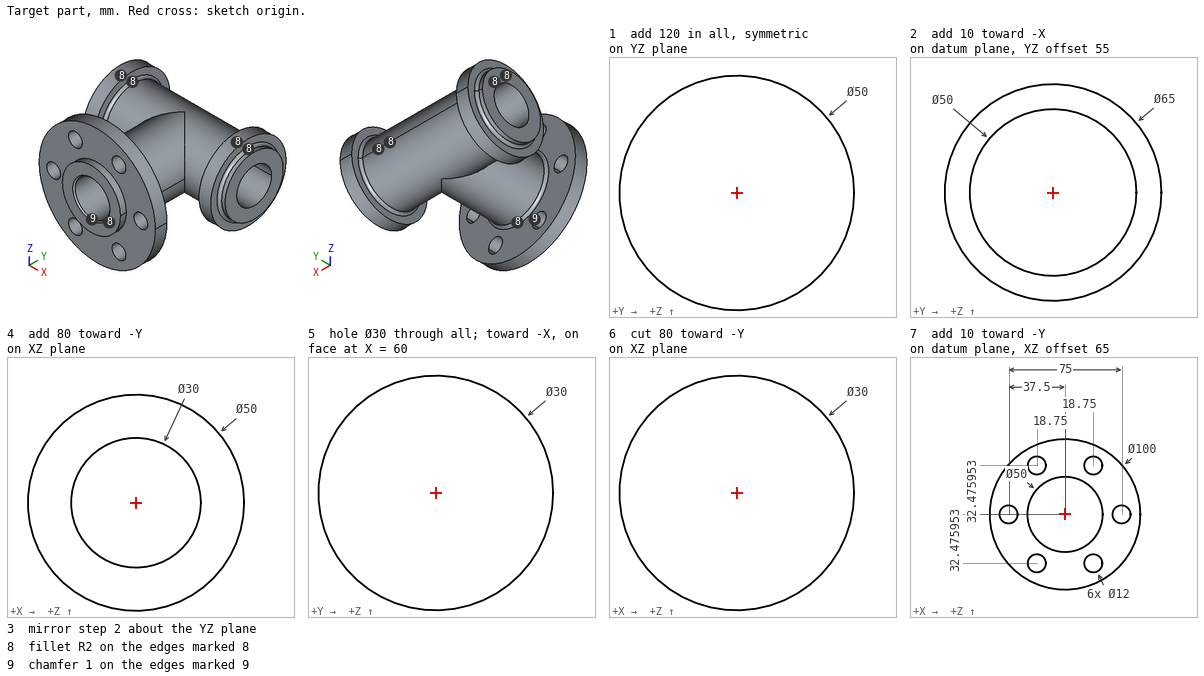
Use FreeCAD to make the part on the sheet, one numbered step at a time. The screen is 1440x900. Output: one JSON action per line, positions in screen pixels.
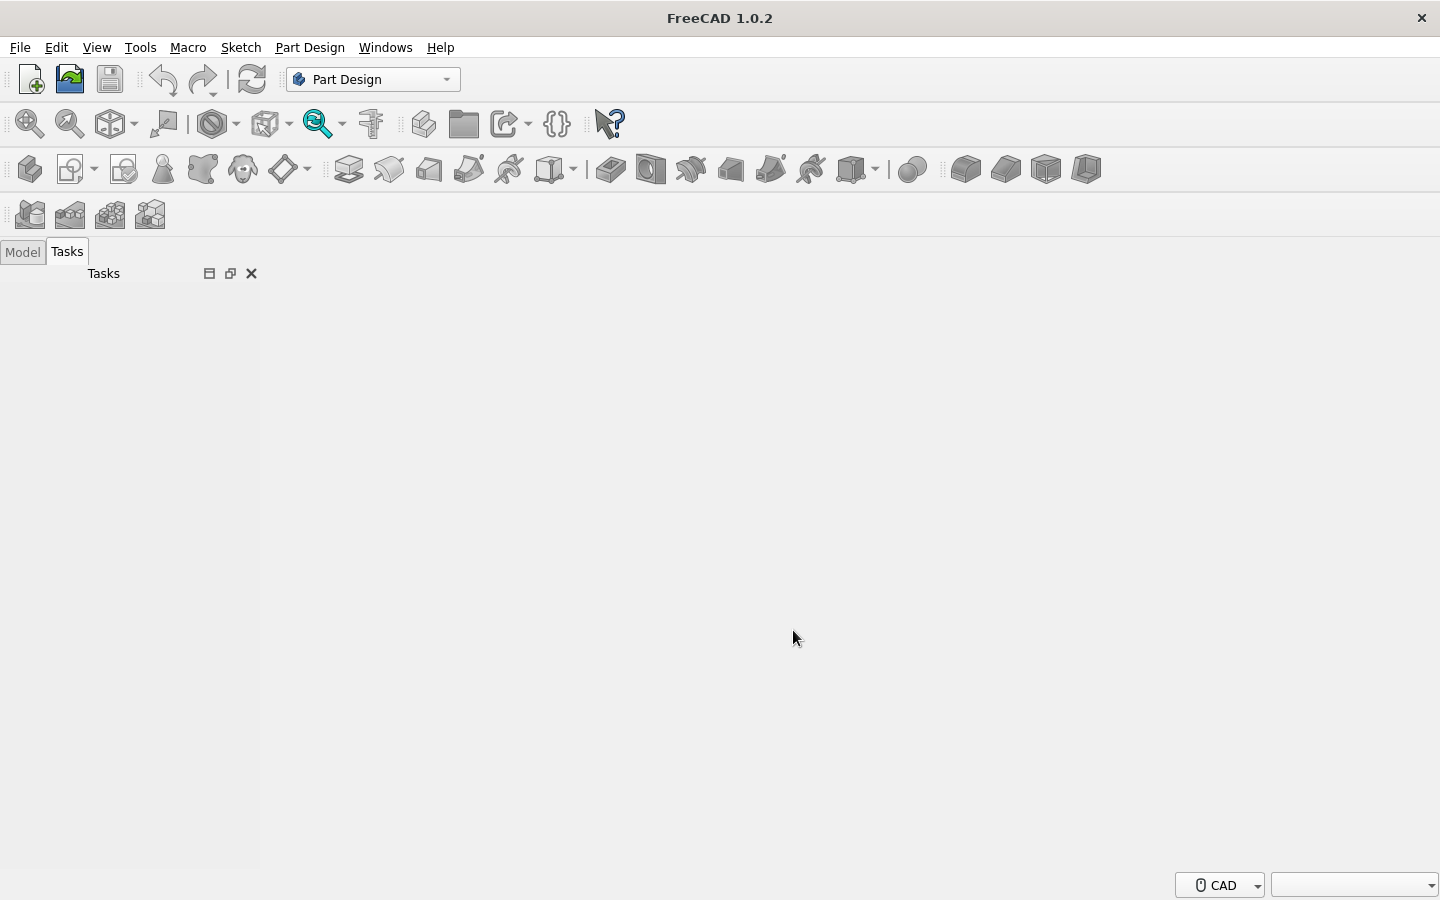
{"action": "key", "text": "ctrl+n"}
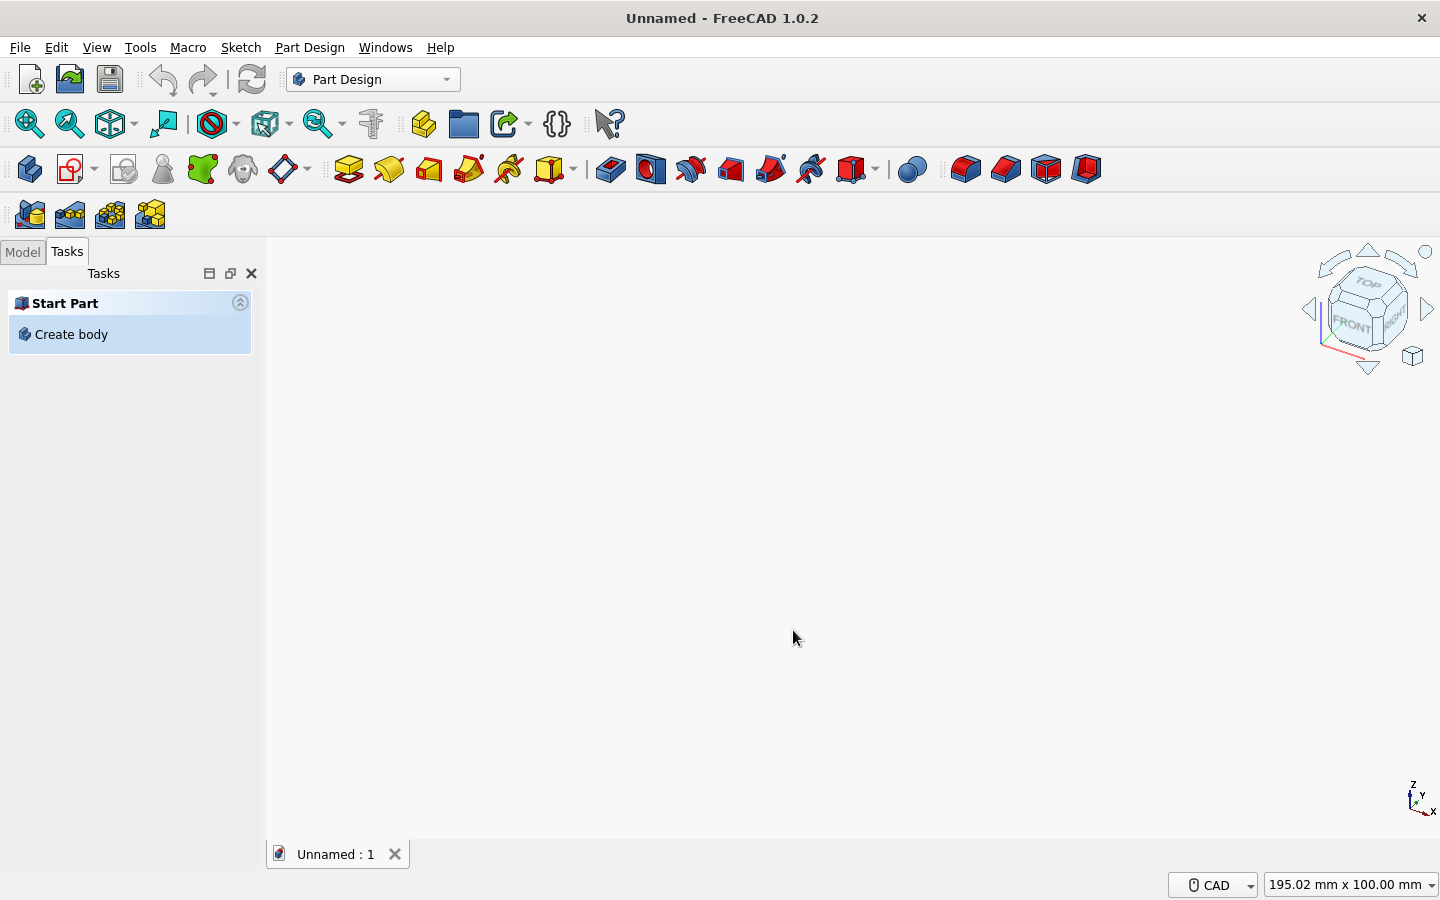
{"action": "left_click", "coordinate": [70, 170]}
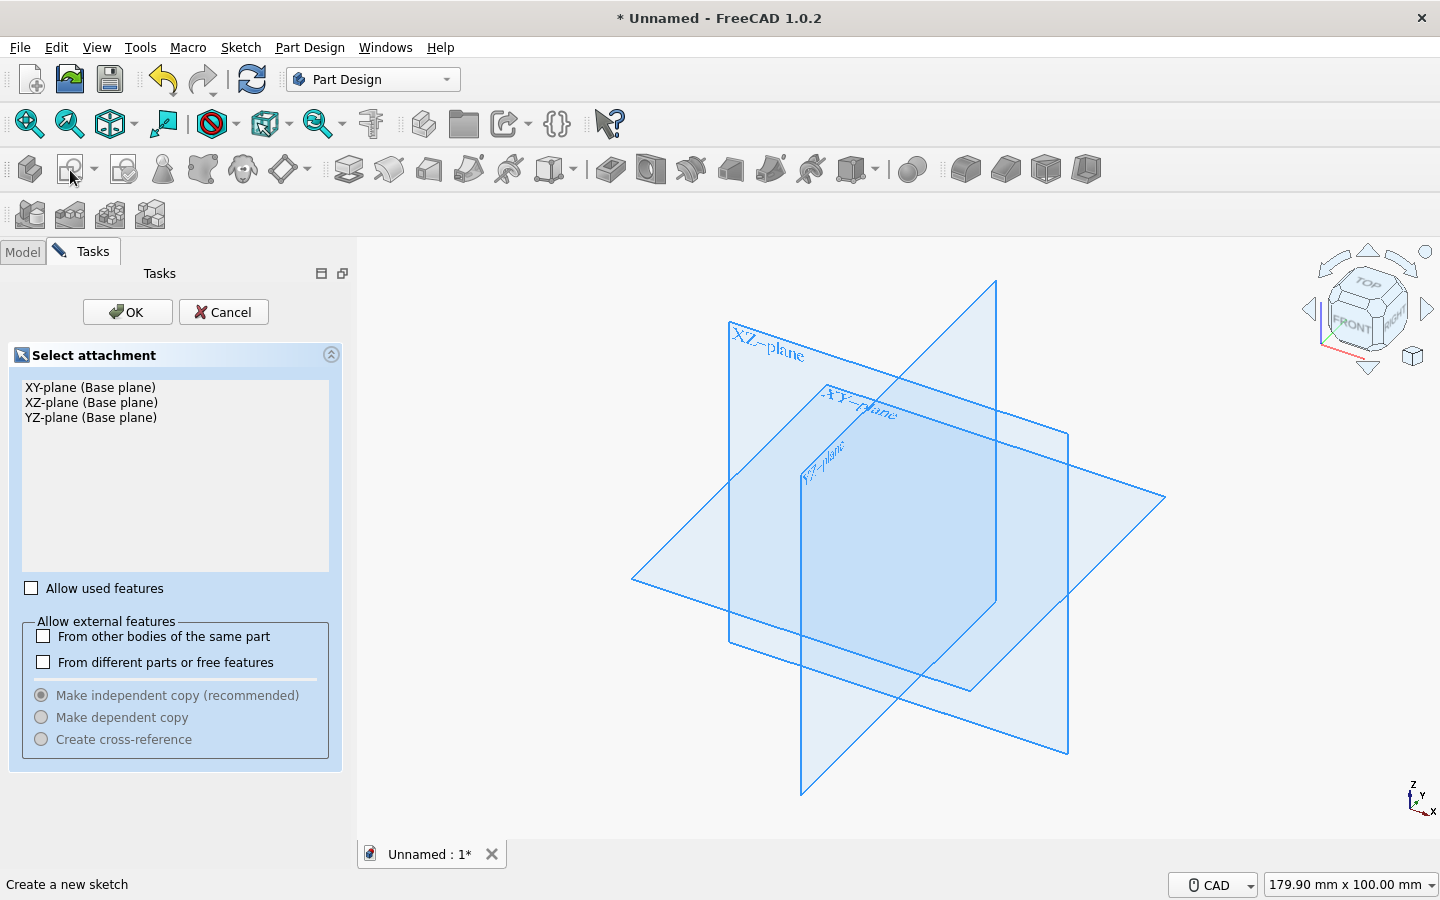
{"action": "left_click", "coordinate": [82, 418]}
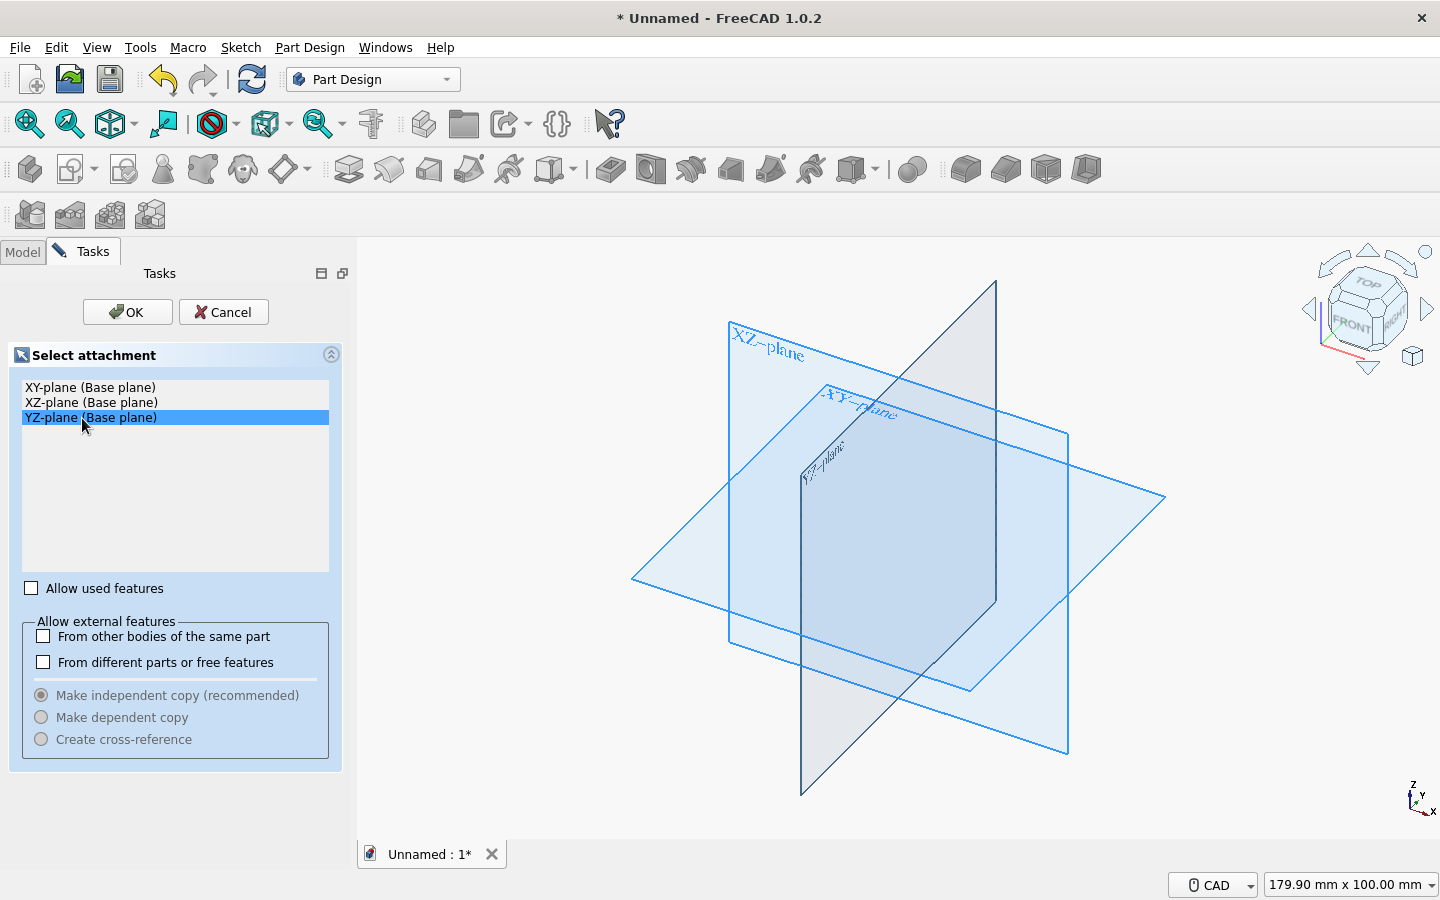
{"action": "left_click", "coordinate": [128, 312]}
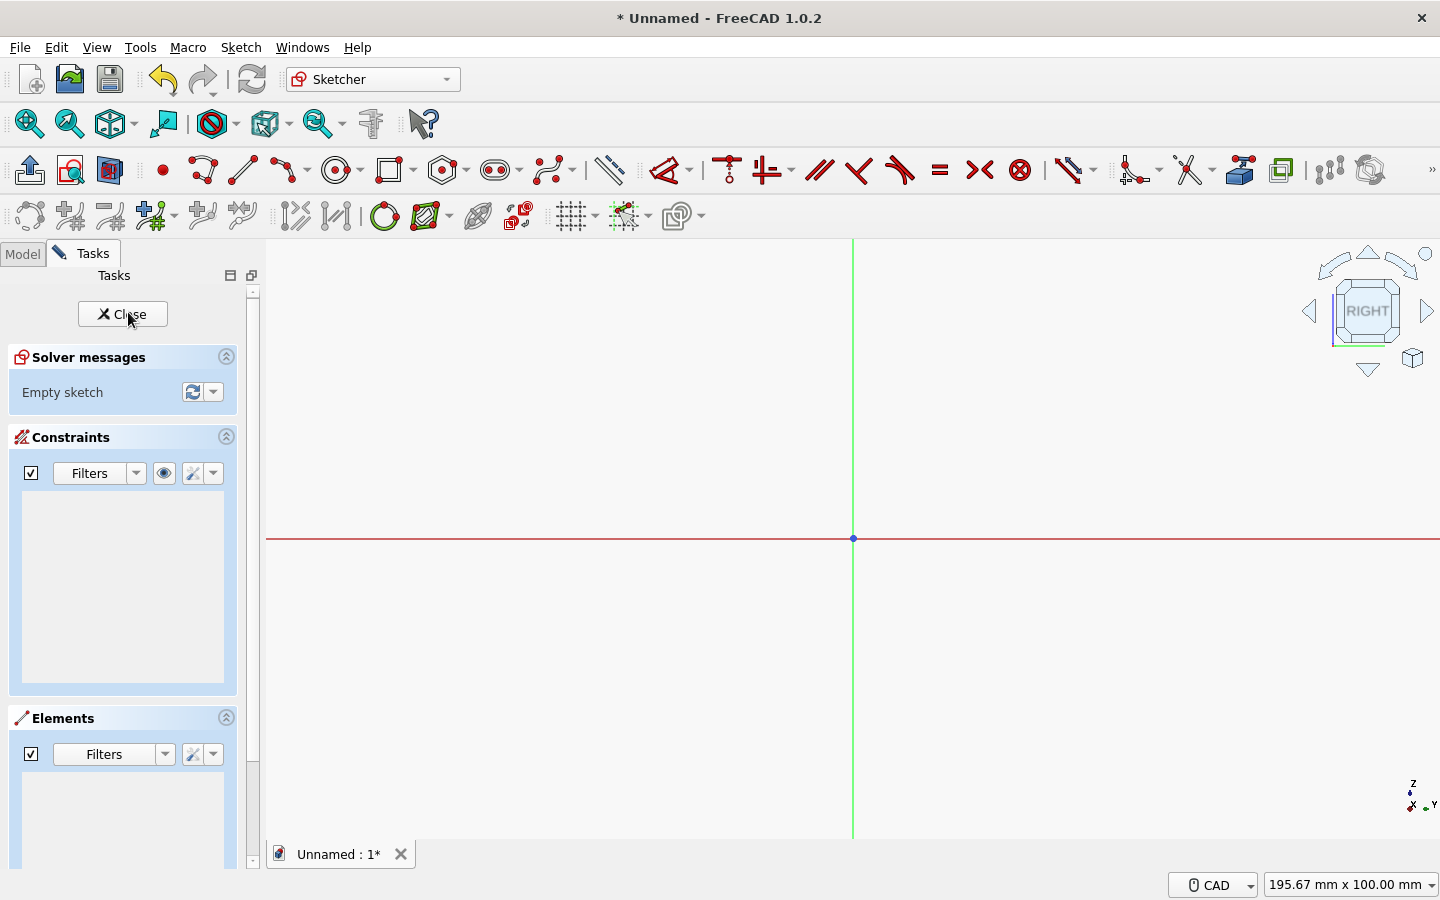
{"action": "left_click", "coordinate": [336, 170]}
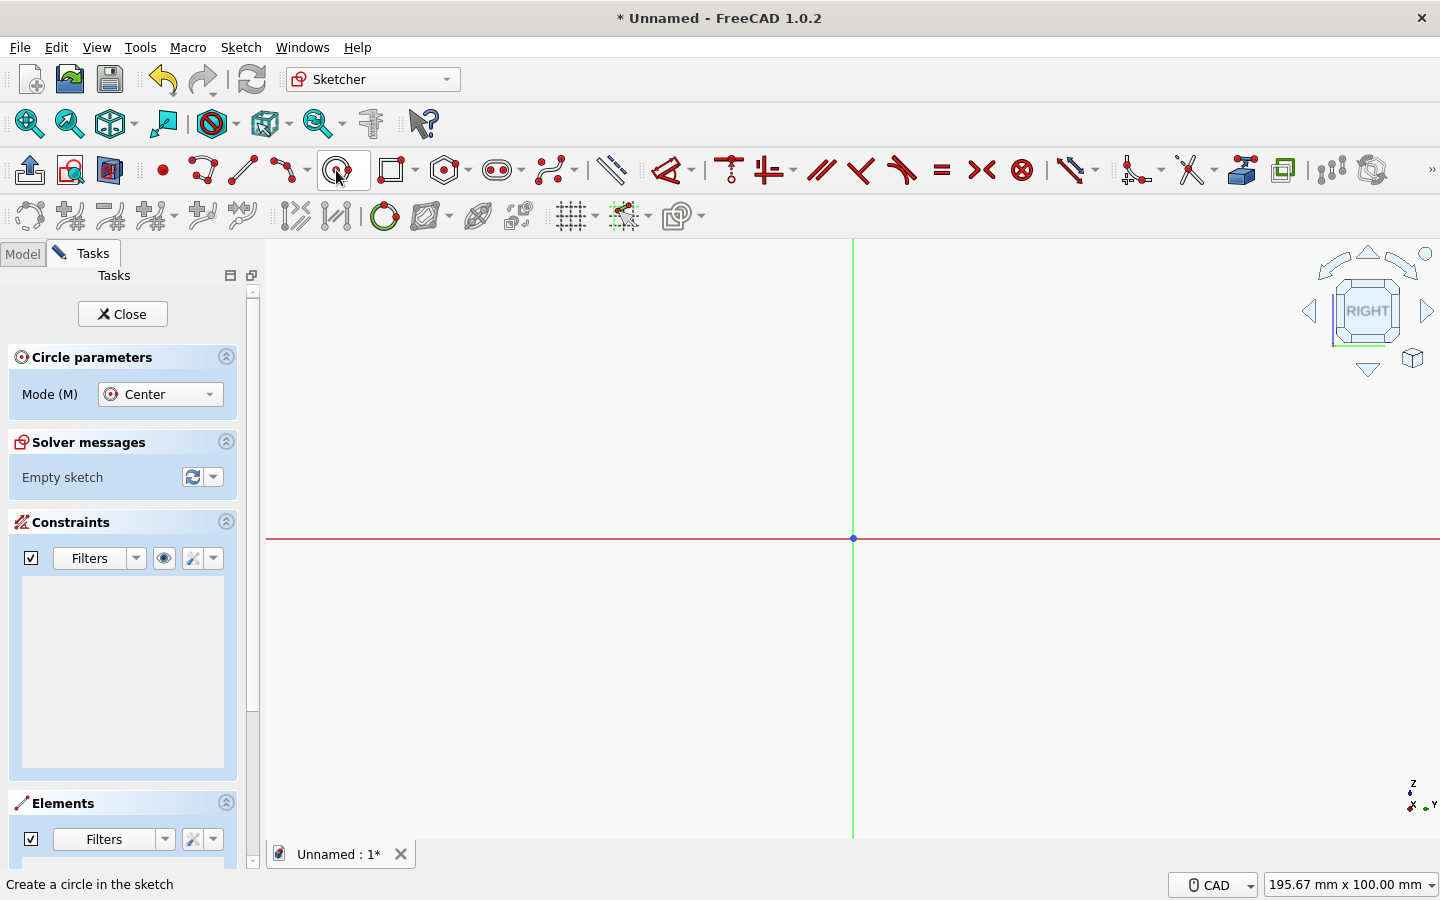
{"action": "left_click", "coordinate": [853, 539]}
{"action": "left_click", "coordinate": [959, 433]}
{"action": "key", "text": "Escape"}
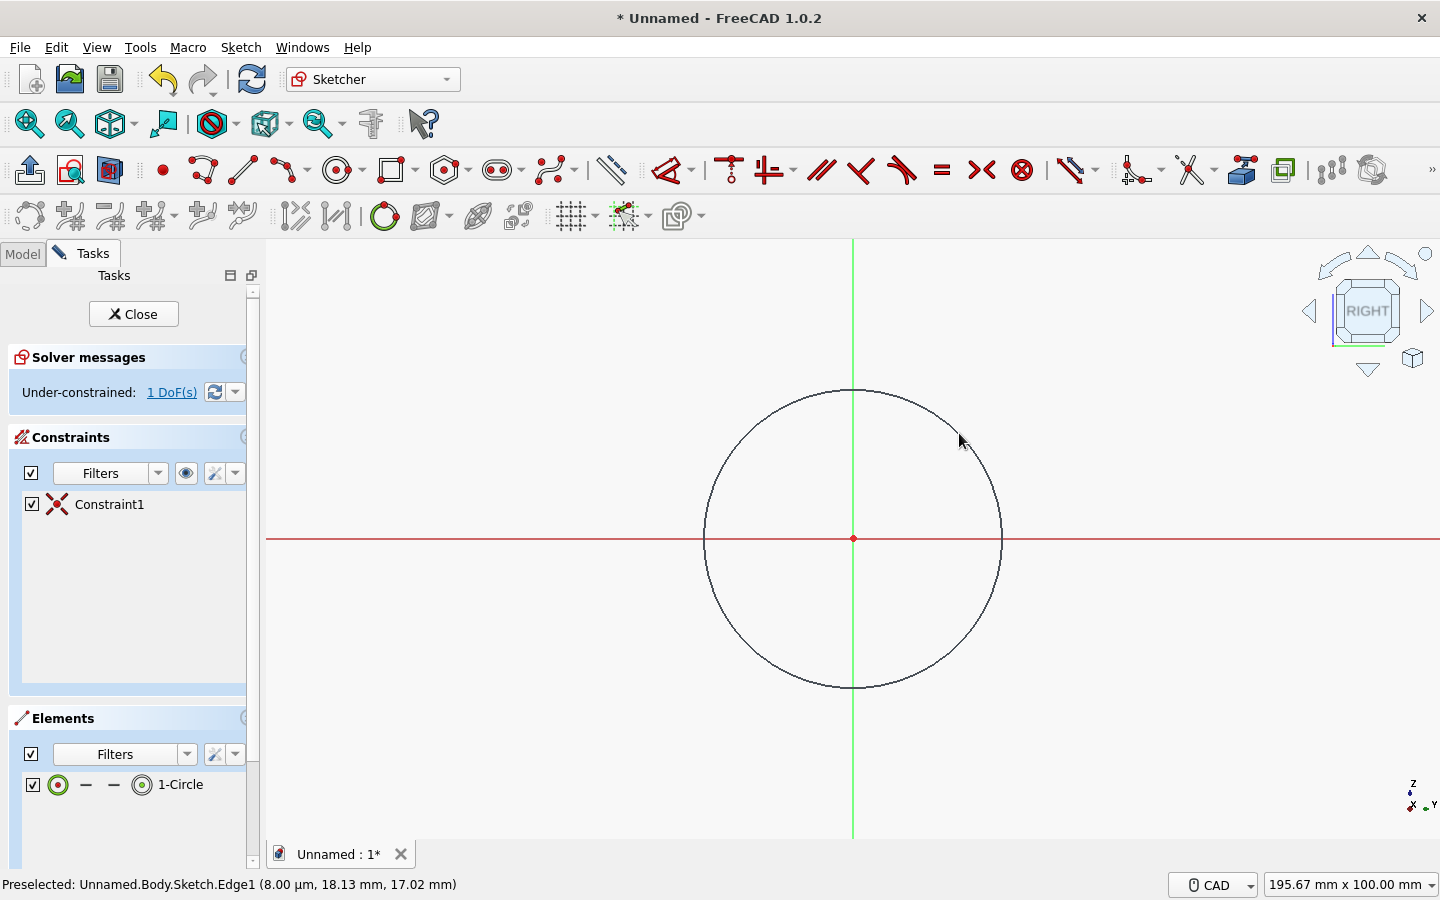
{"action": "left_click", "coordinate": [958, 433]}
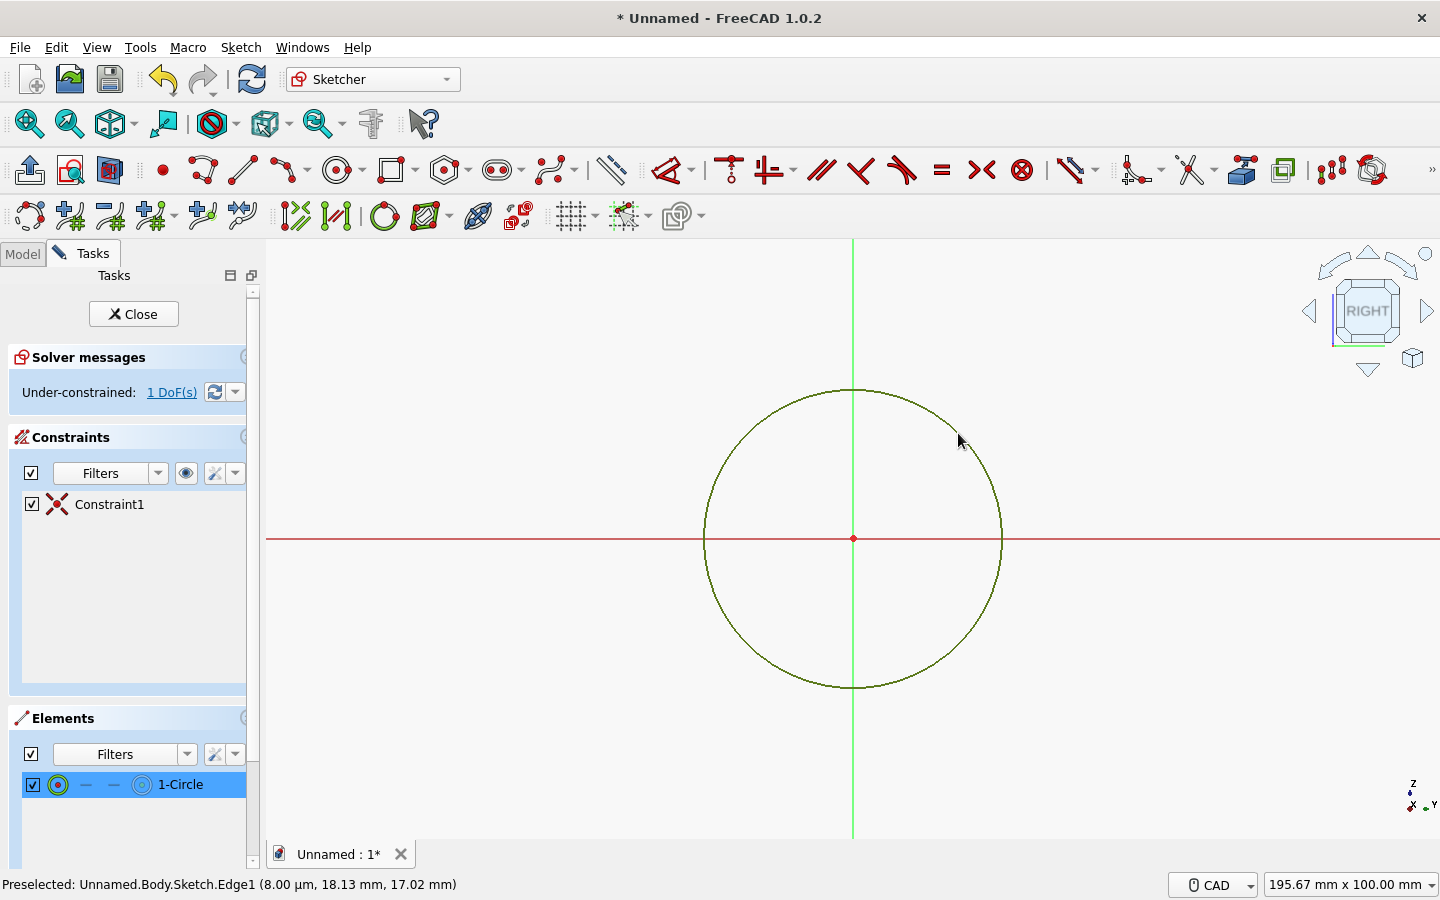
{"action": "key", "text": "k o"}